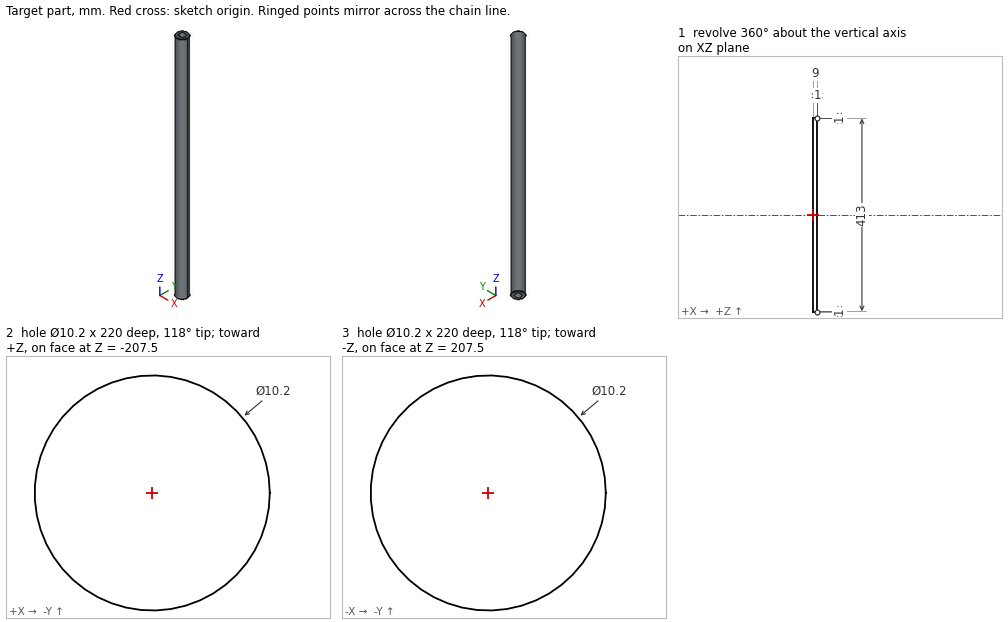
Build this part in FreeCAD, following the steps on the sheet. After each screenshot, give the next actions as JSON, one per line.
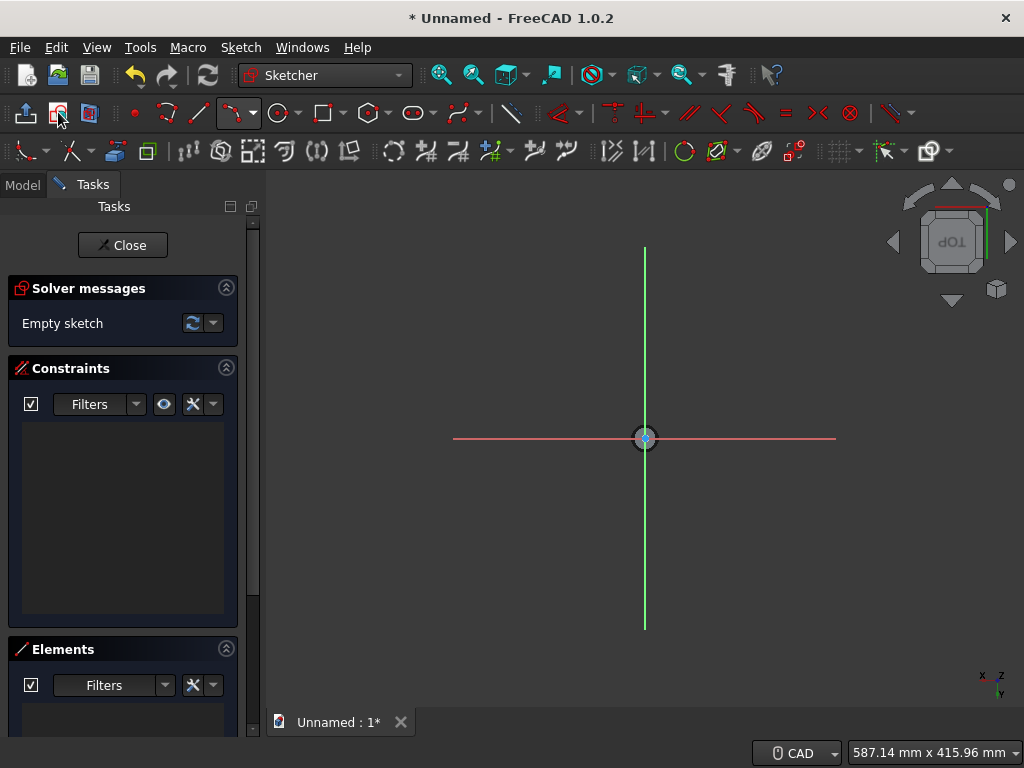
{"action": "scroll", "coordinate": [649, 439], "scroll_direction": "up", "scroll_amount": 15}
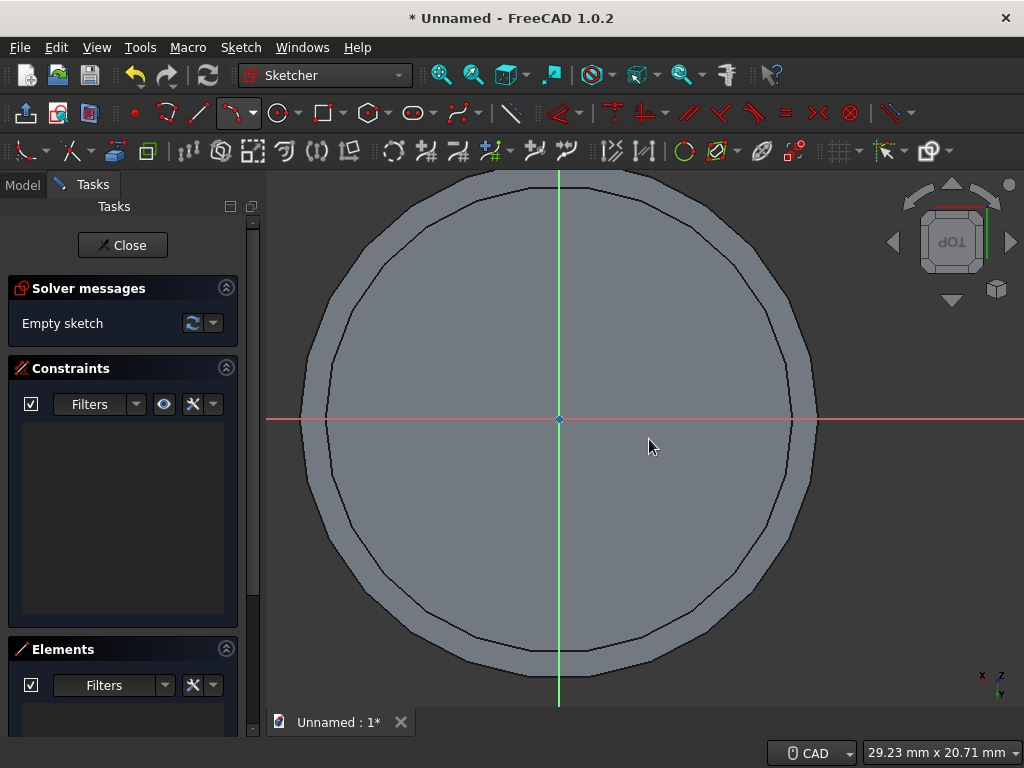
{"action": "key", "text": "g c"}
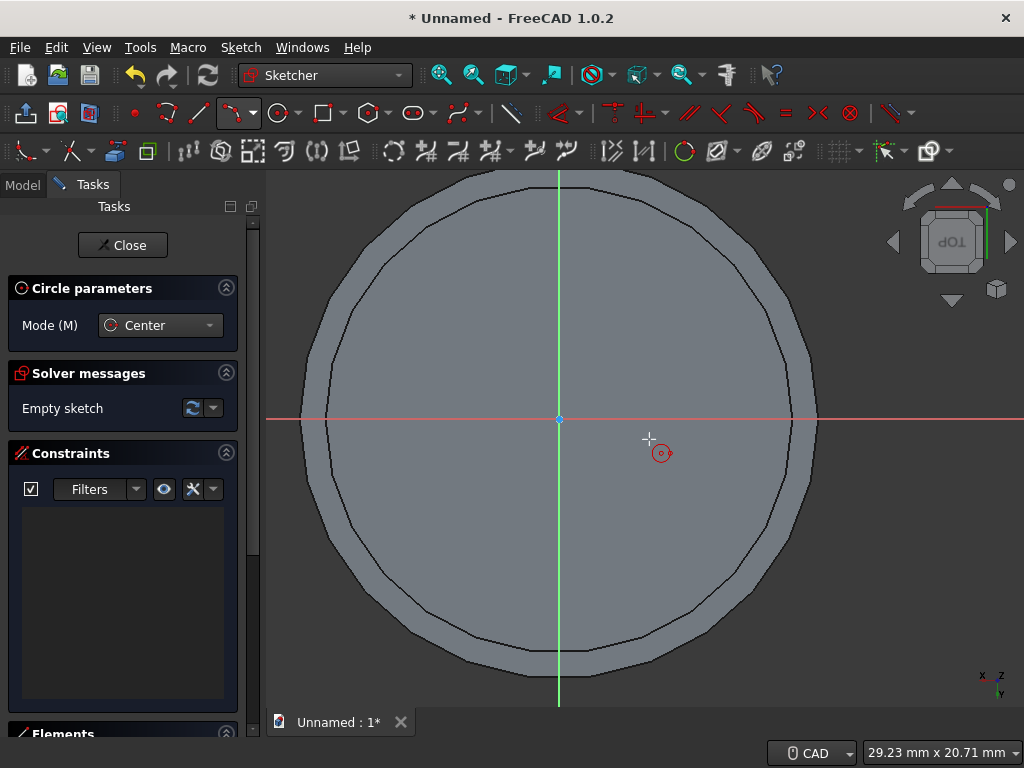
{"action": "left_click", "coordinate": [559, 419]}
{"action": "left_click", "coordinate": [653, 326]}
{"action": "key", "text": "Escape"}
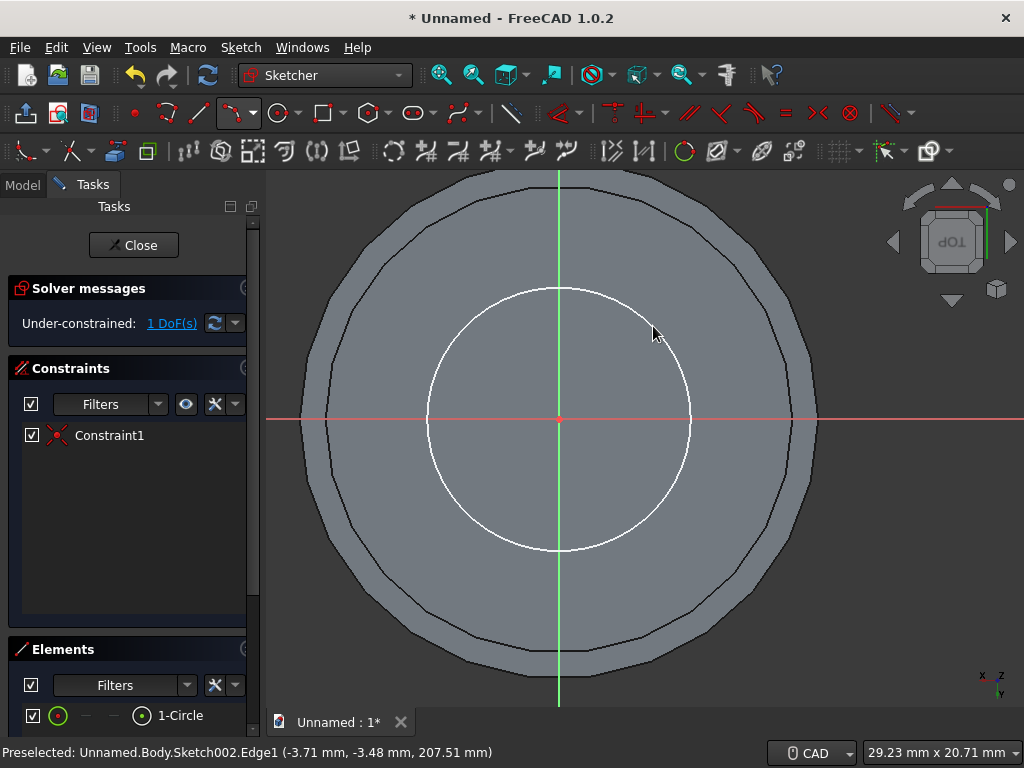
{"action": "left_click", "coordinate": [558, 114]}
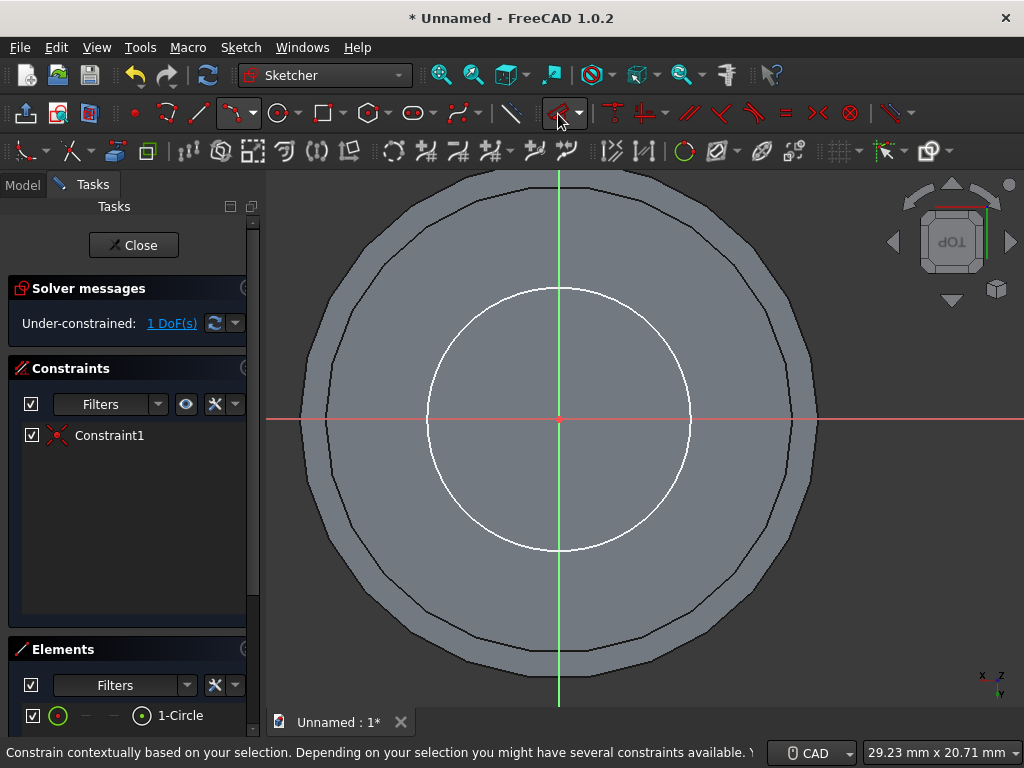
{"action": "left_click", "coordinate": [652, 326]}
{"action": "left_click", "coordinate": [675, 303]}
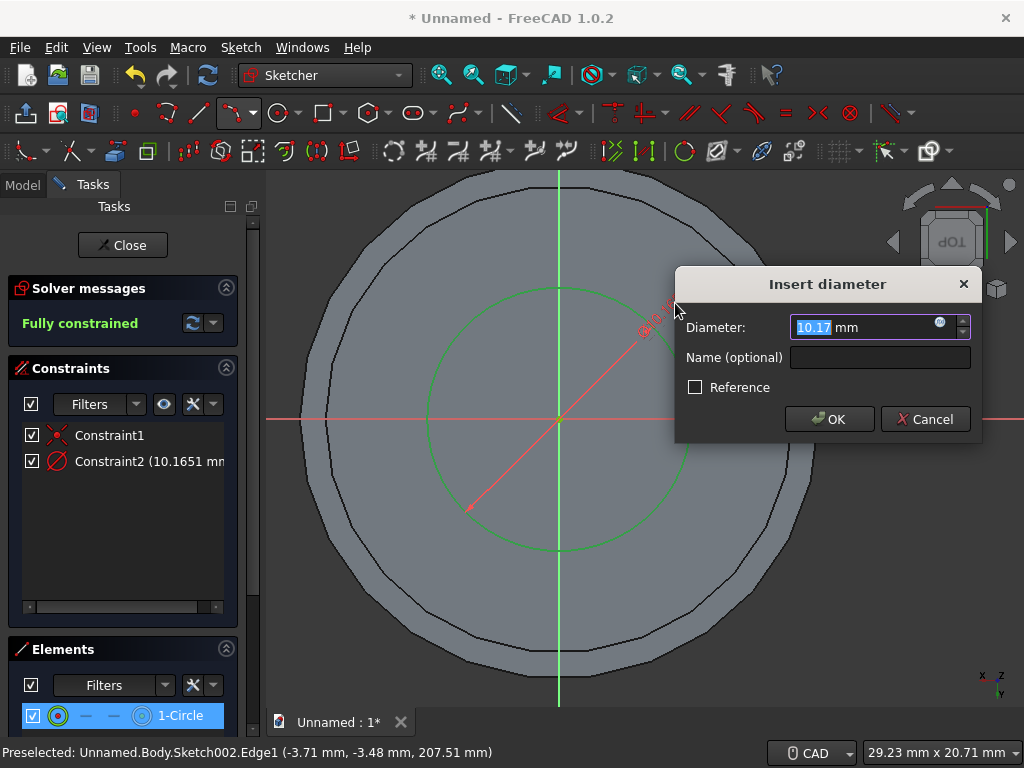
{"action": "type", "text": "10.2"}
{"action": "key", "text": "Return"}
{"action": "key", "text": "Escape"}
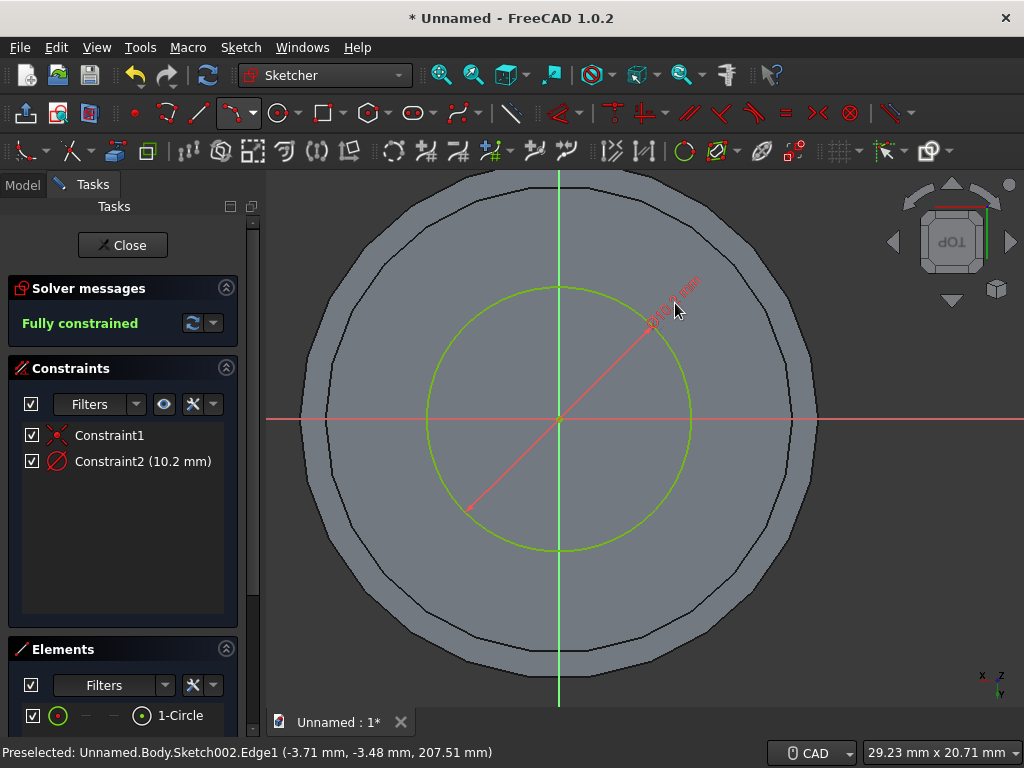
{"action": "left_click", "coordinate": [123, 245]}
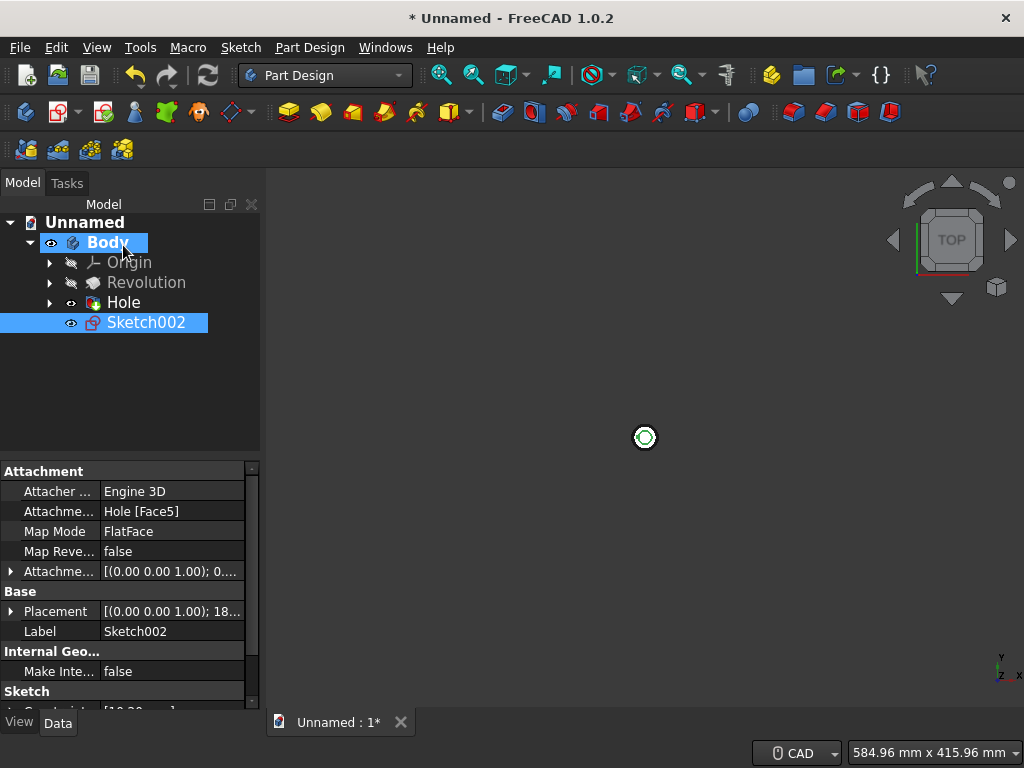
{"action": "left_click", "coordinate": [536, 112]}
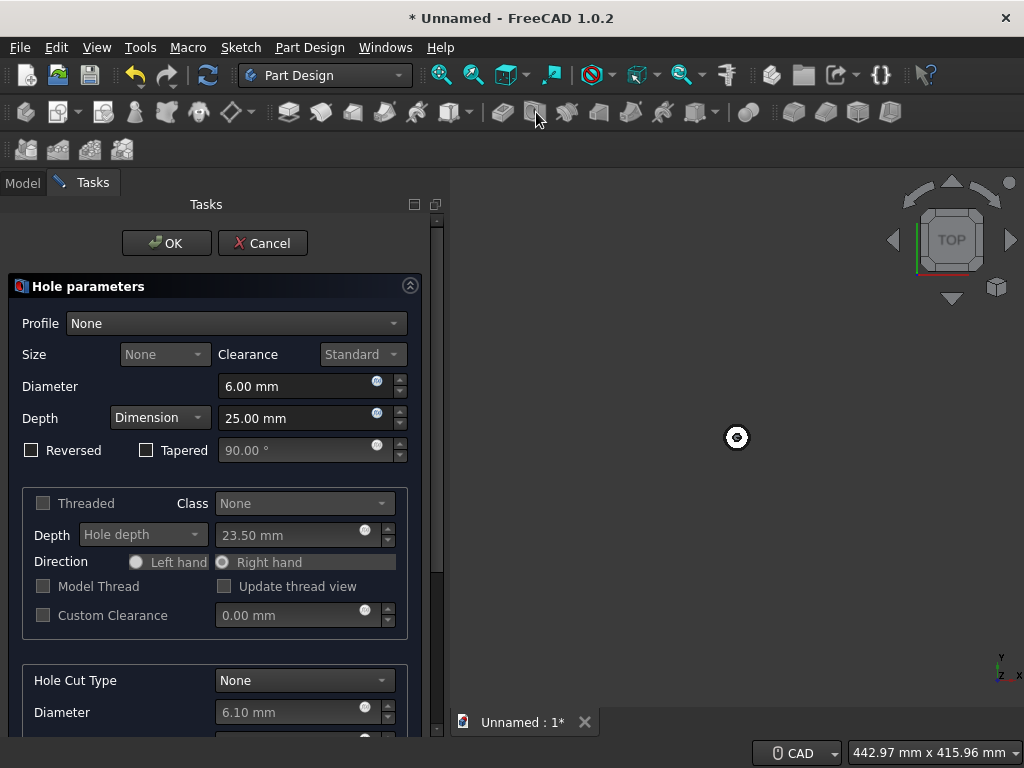
{"action": "triple_click", "coordinate": [305, 386]}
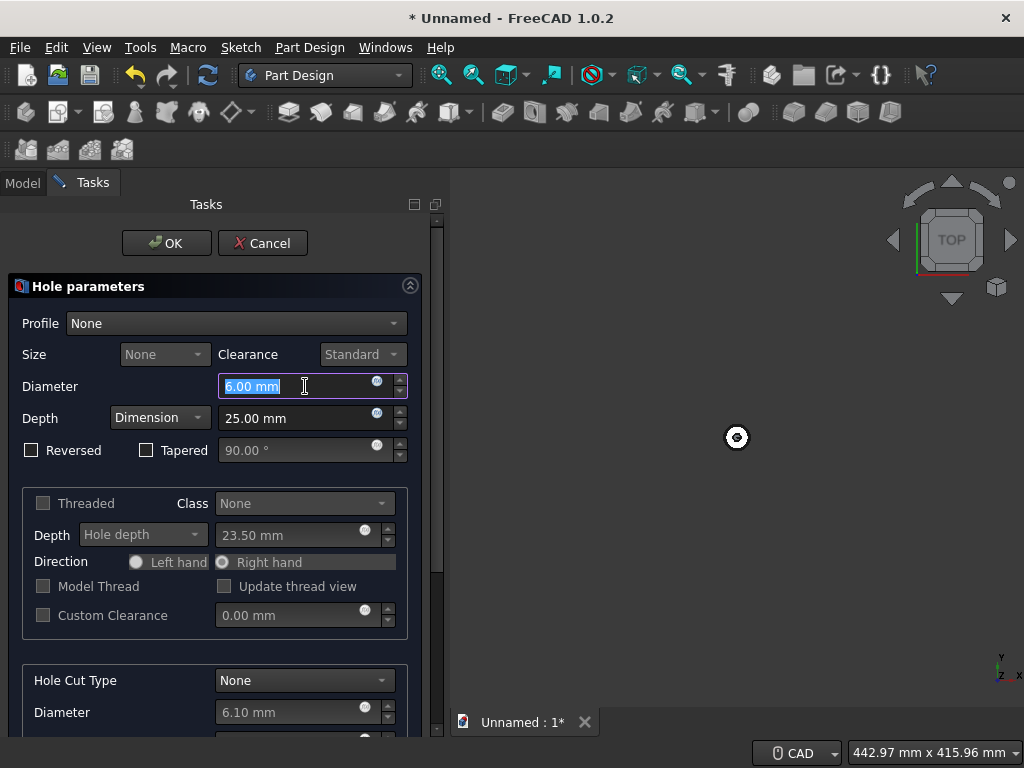
{"action": "type", "text": "10.2"}
{"action": "key", "text": "Tab"}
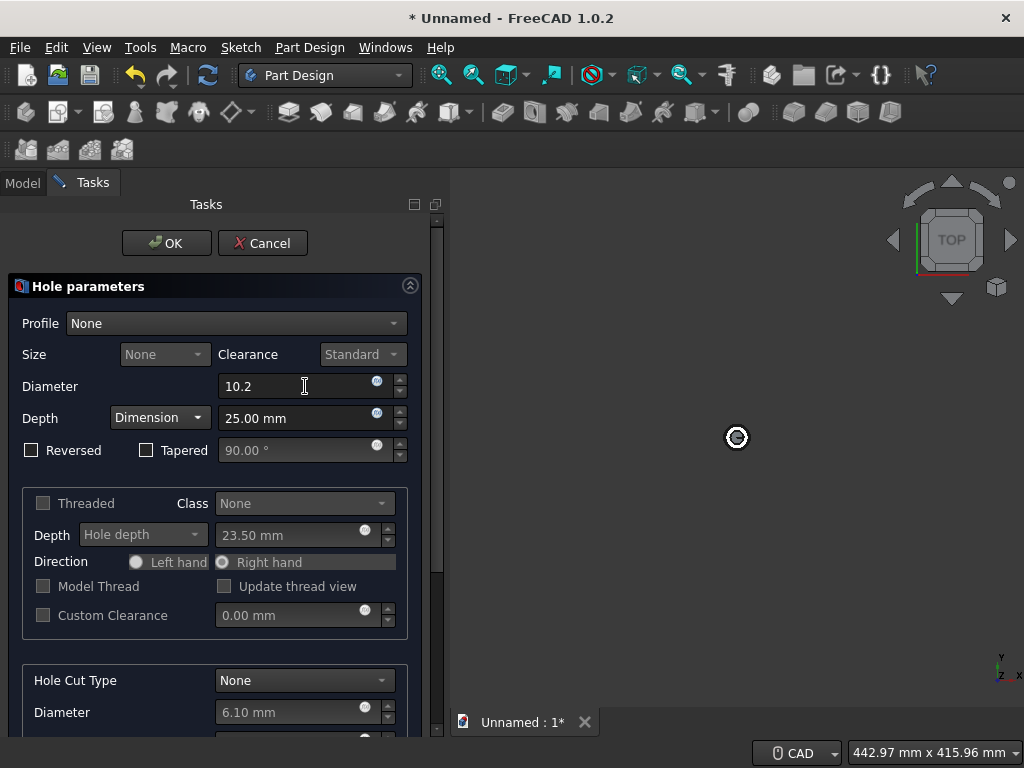
{"action": "triple_click", "coordinate": [305, 418]}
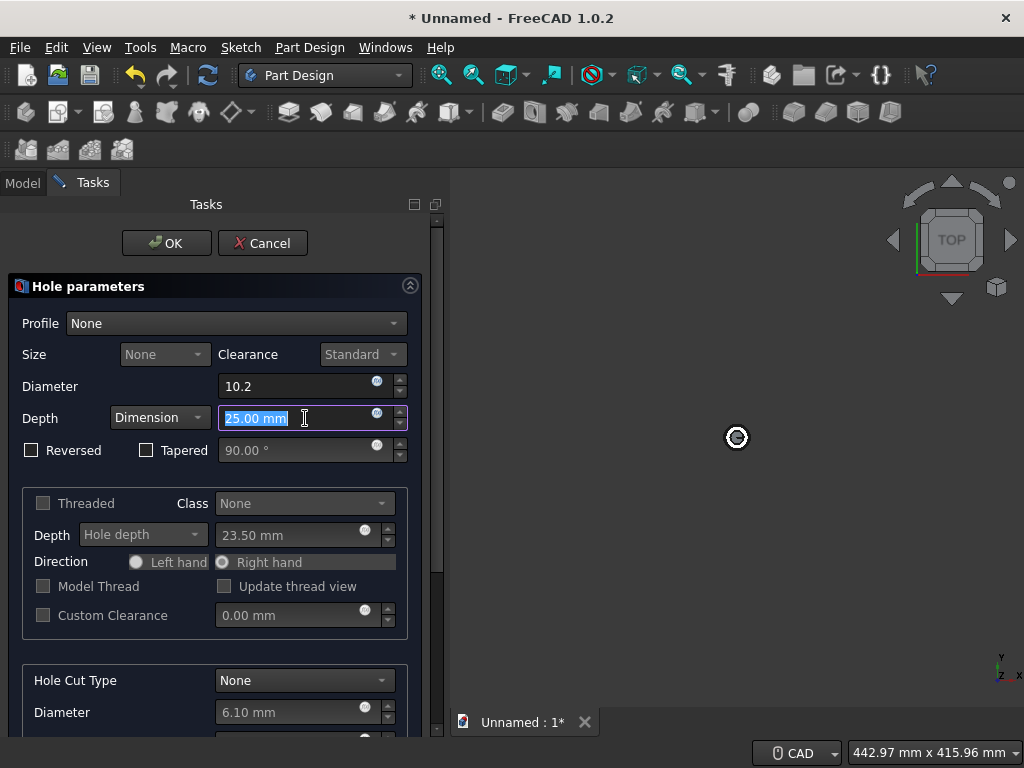
{"action": "type", "text": "220"}
{"action": "key", "text": "Tab"}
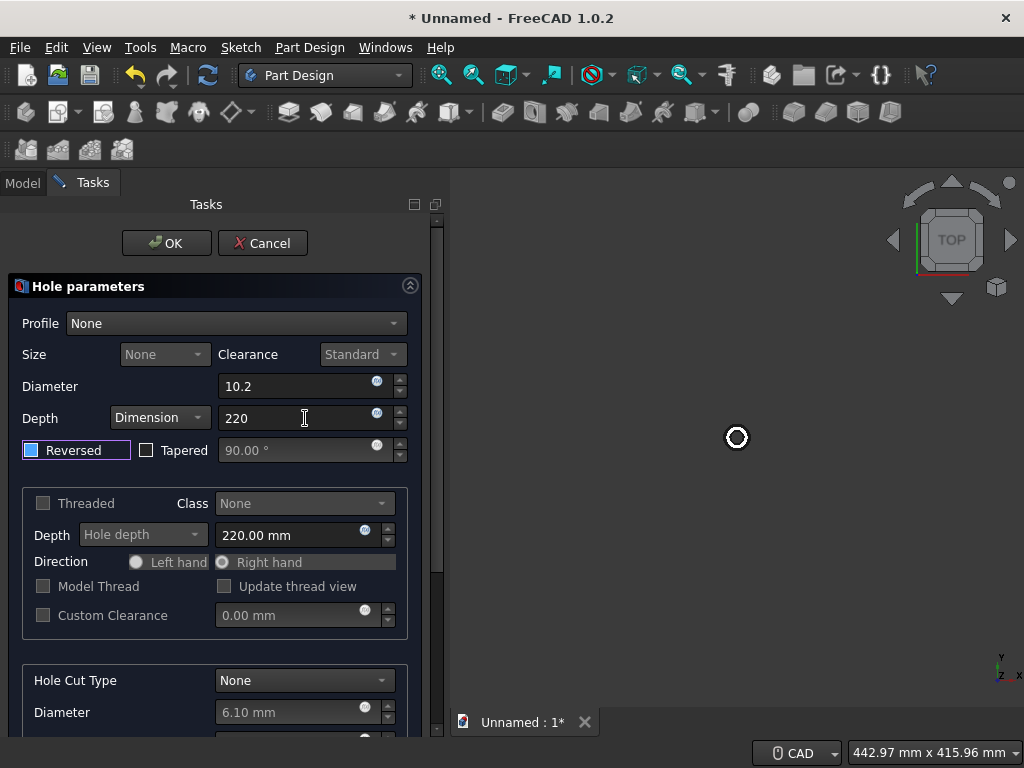
{"action": "left_click", "coordinate": [167, 243]}